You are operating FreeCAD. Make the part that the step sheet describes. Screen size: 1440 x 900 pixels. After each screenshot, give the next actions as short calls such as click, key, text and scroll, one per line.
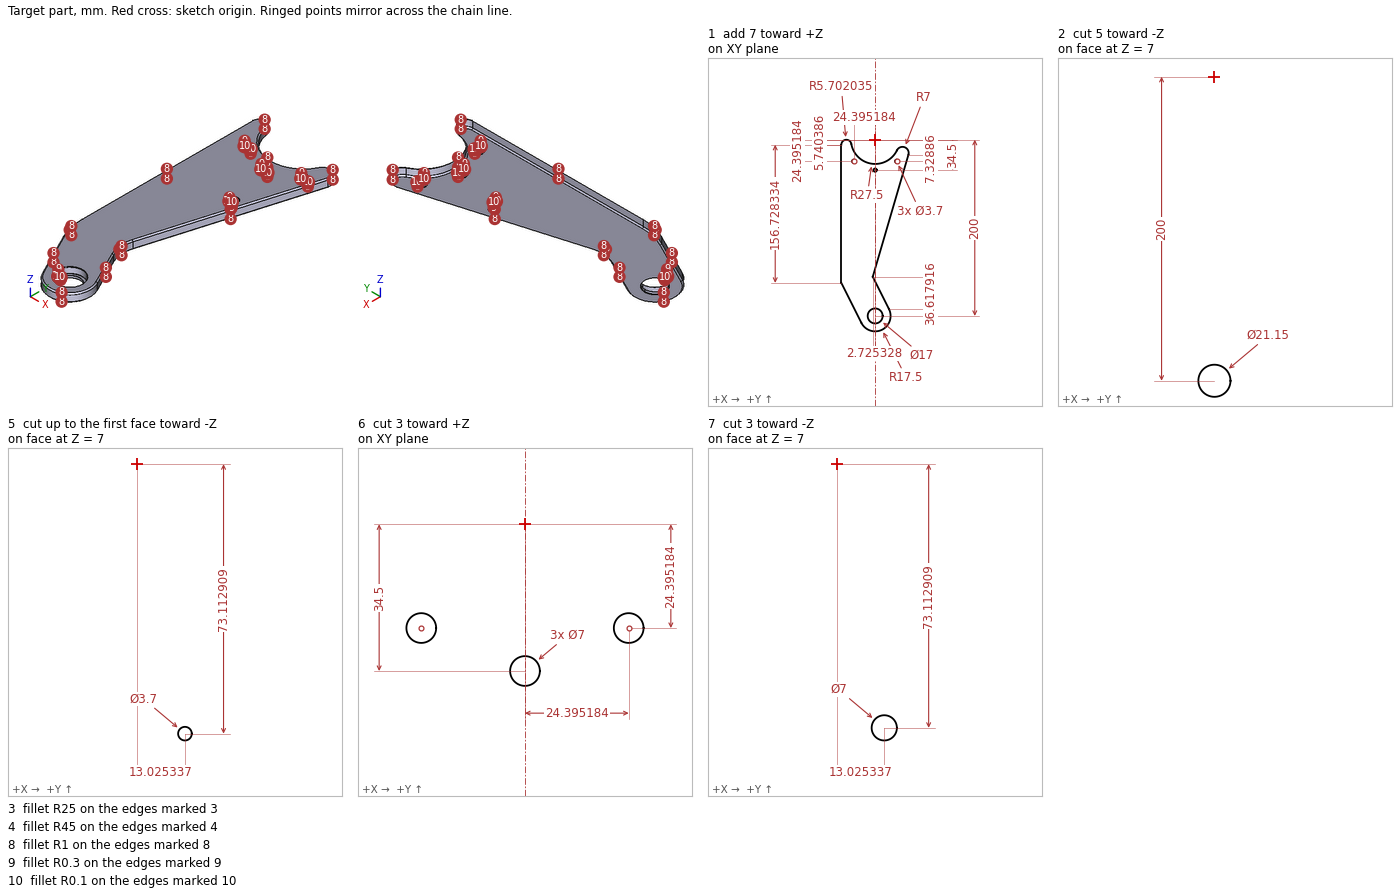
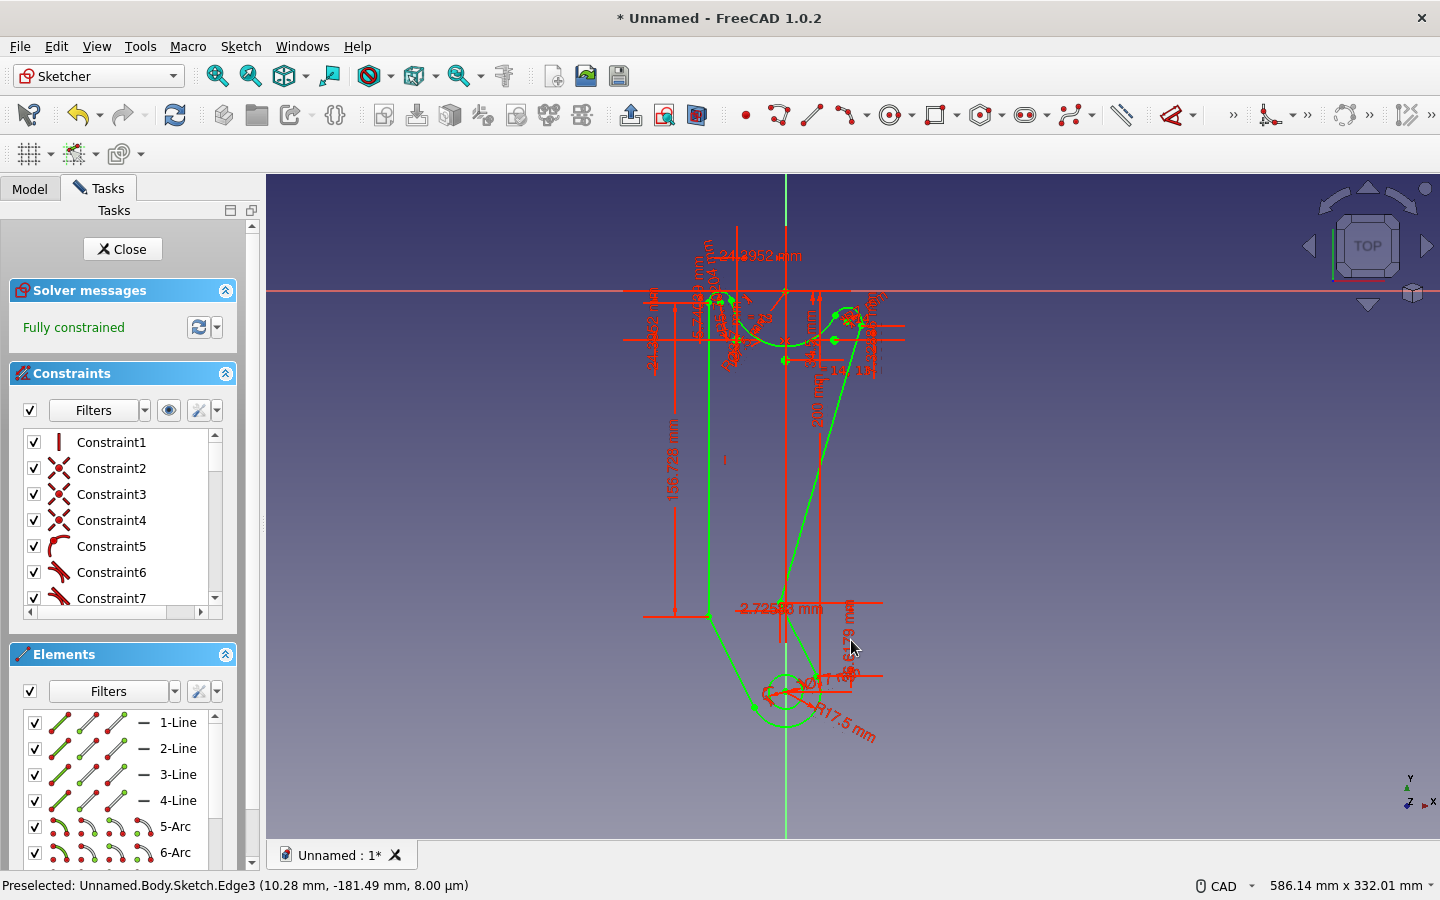
click(123, 249)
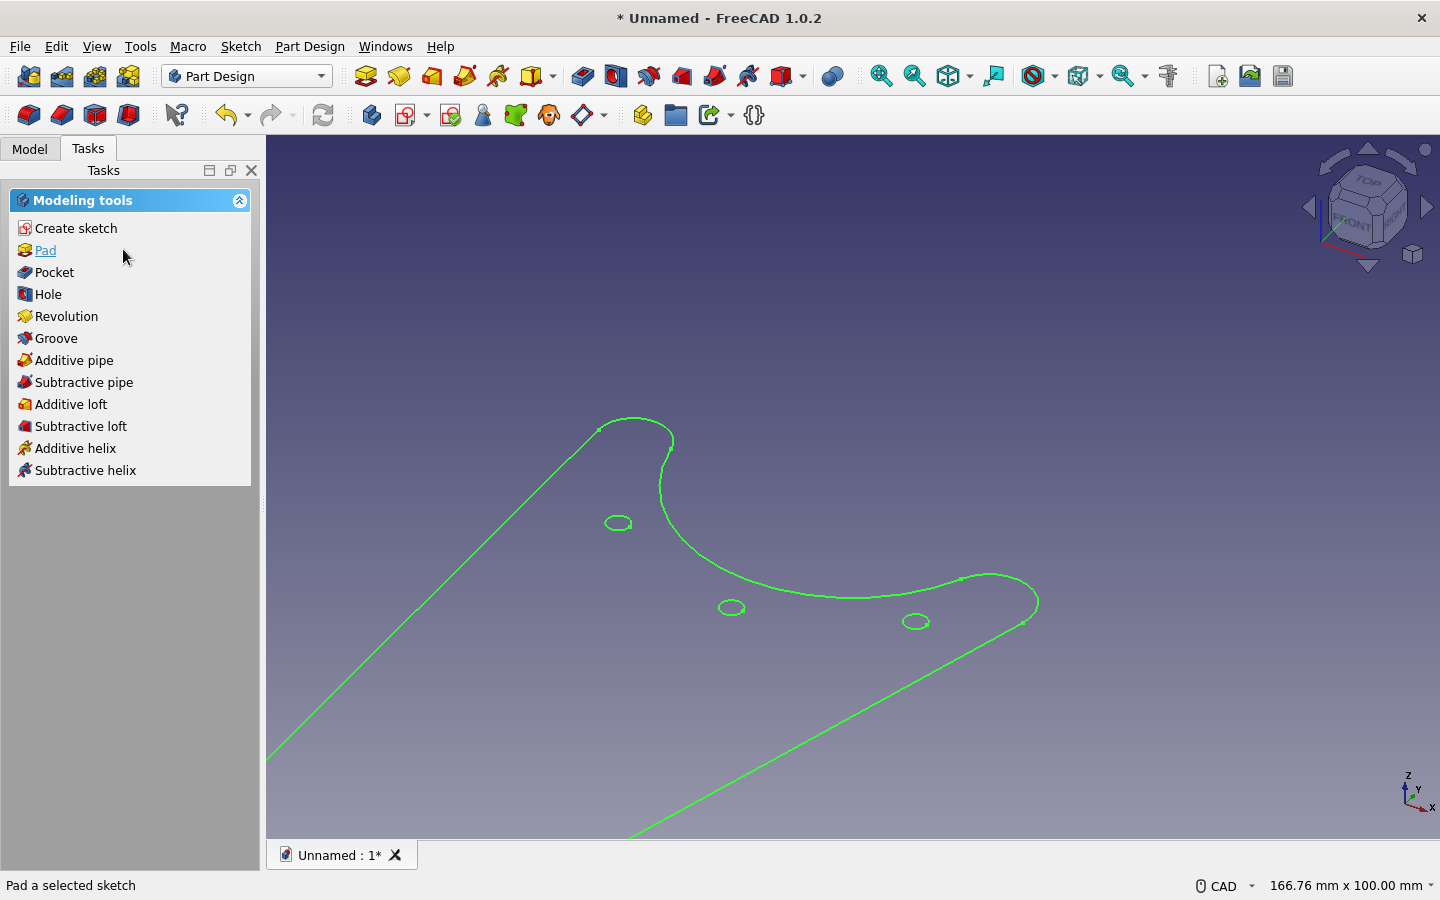
click(366, 76)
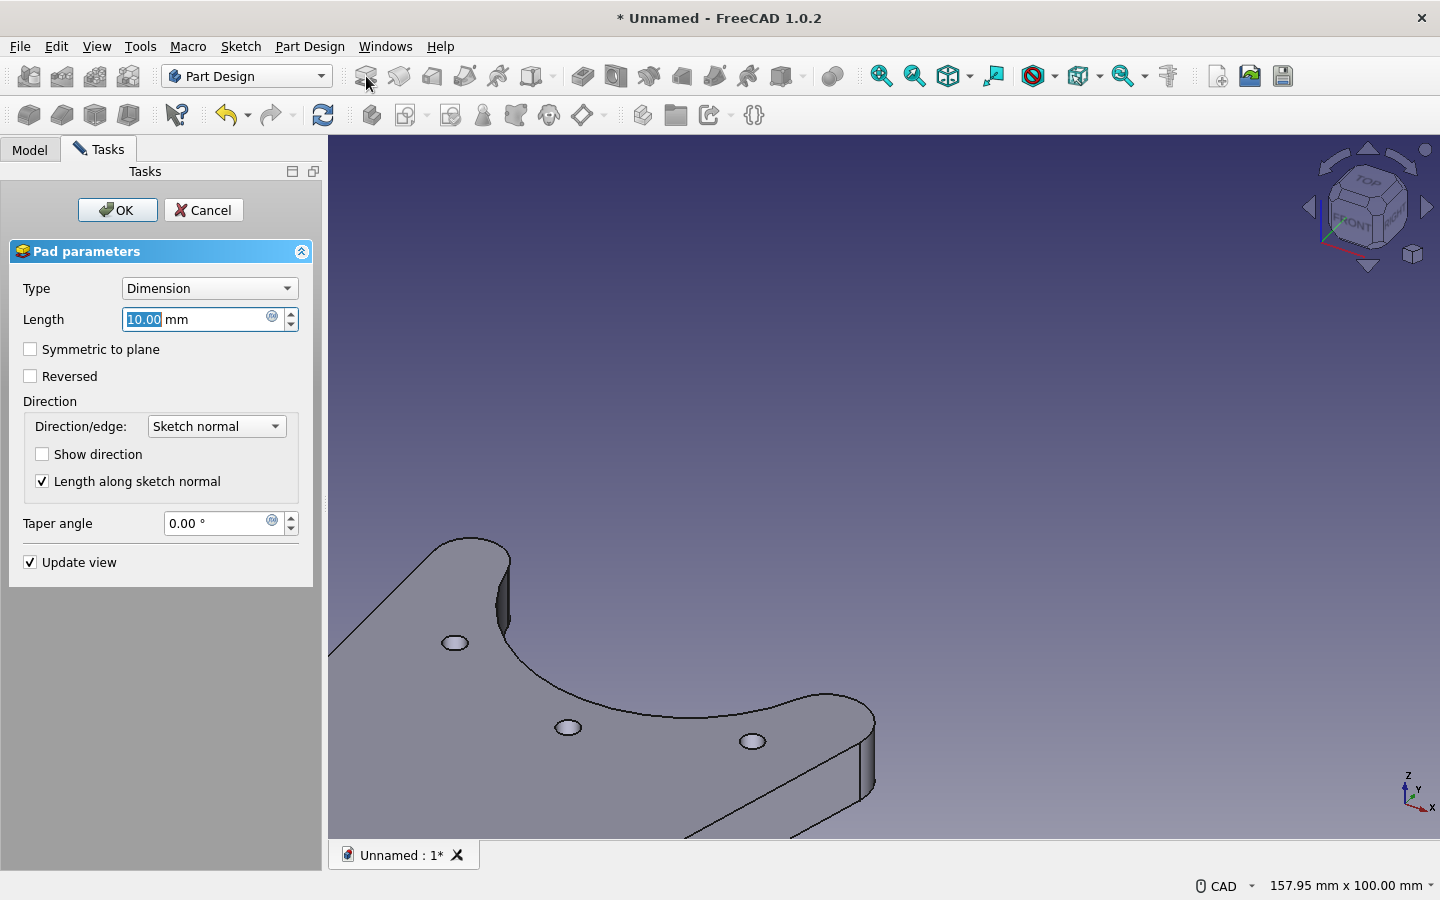
text(7)
key(Tab)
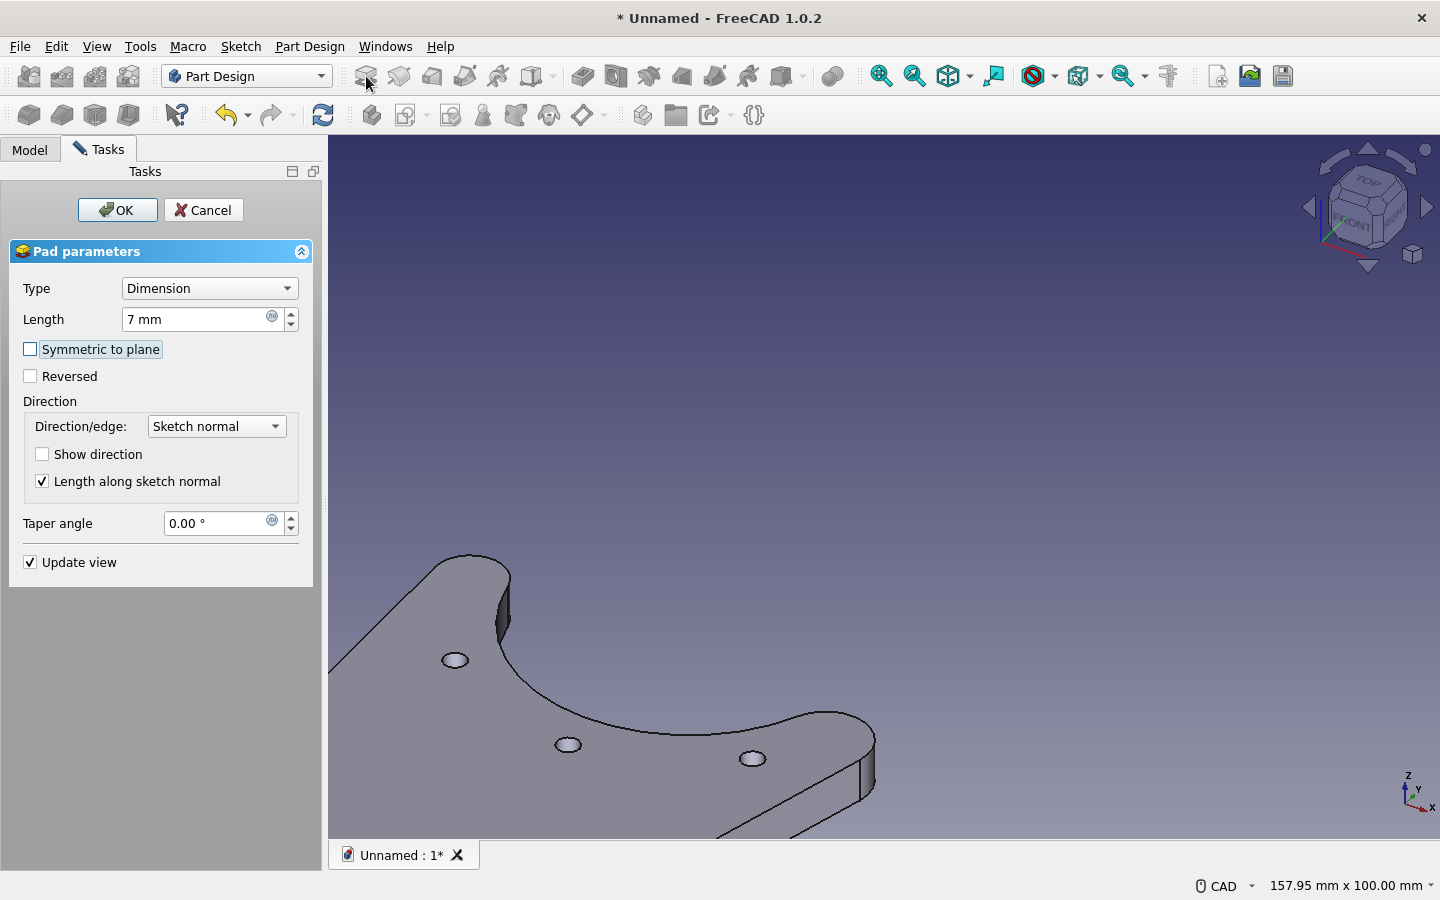
click(118, 210)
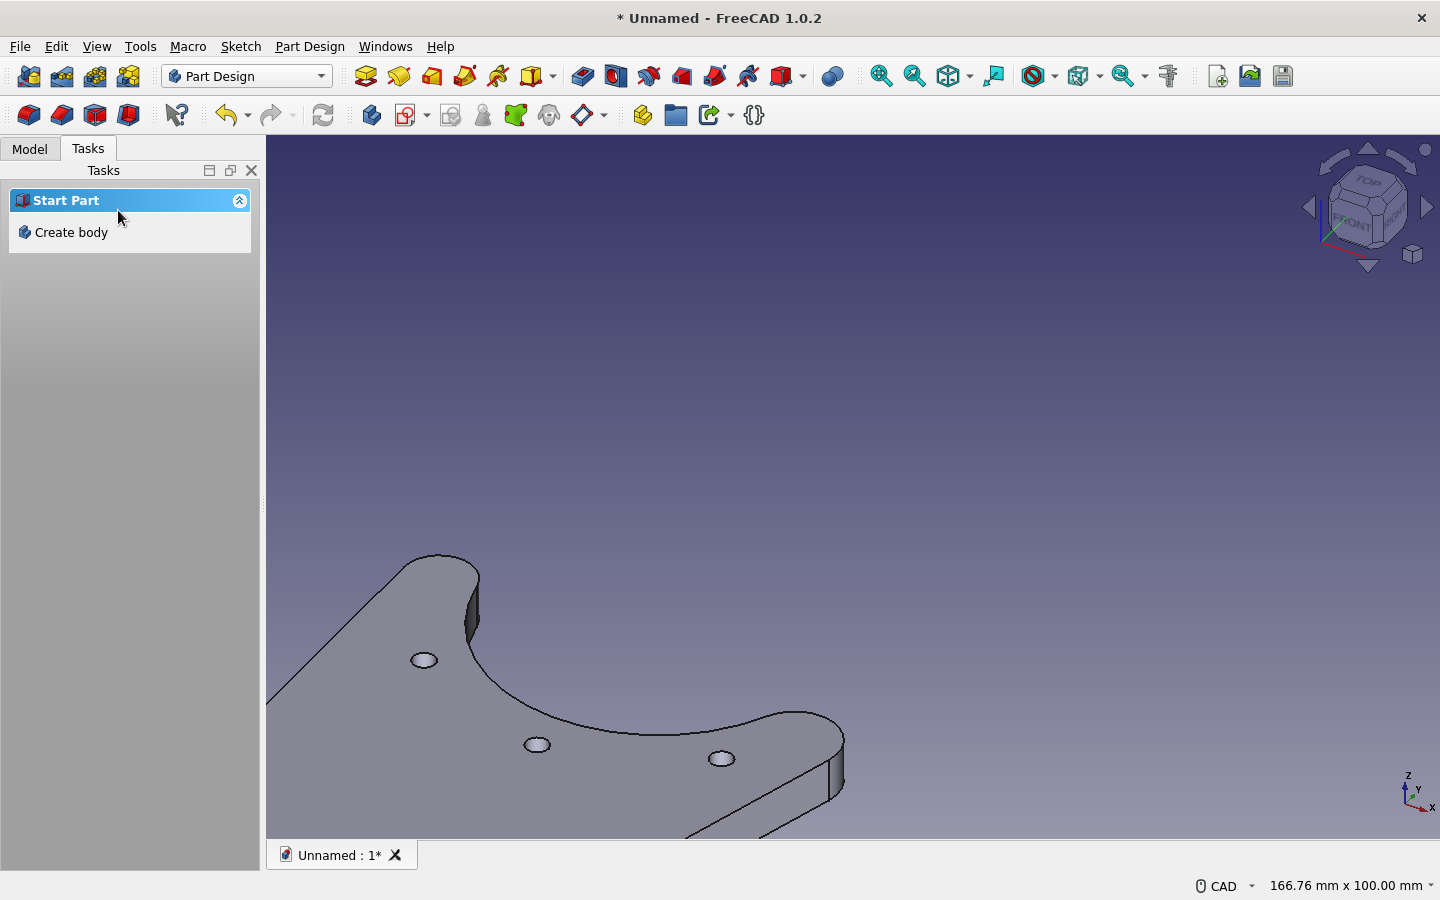
click(882, 76)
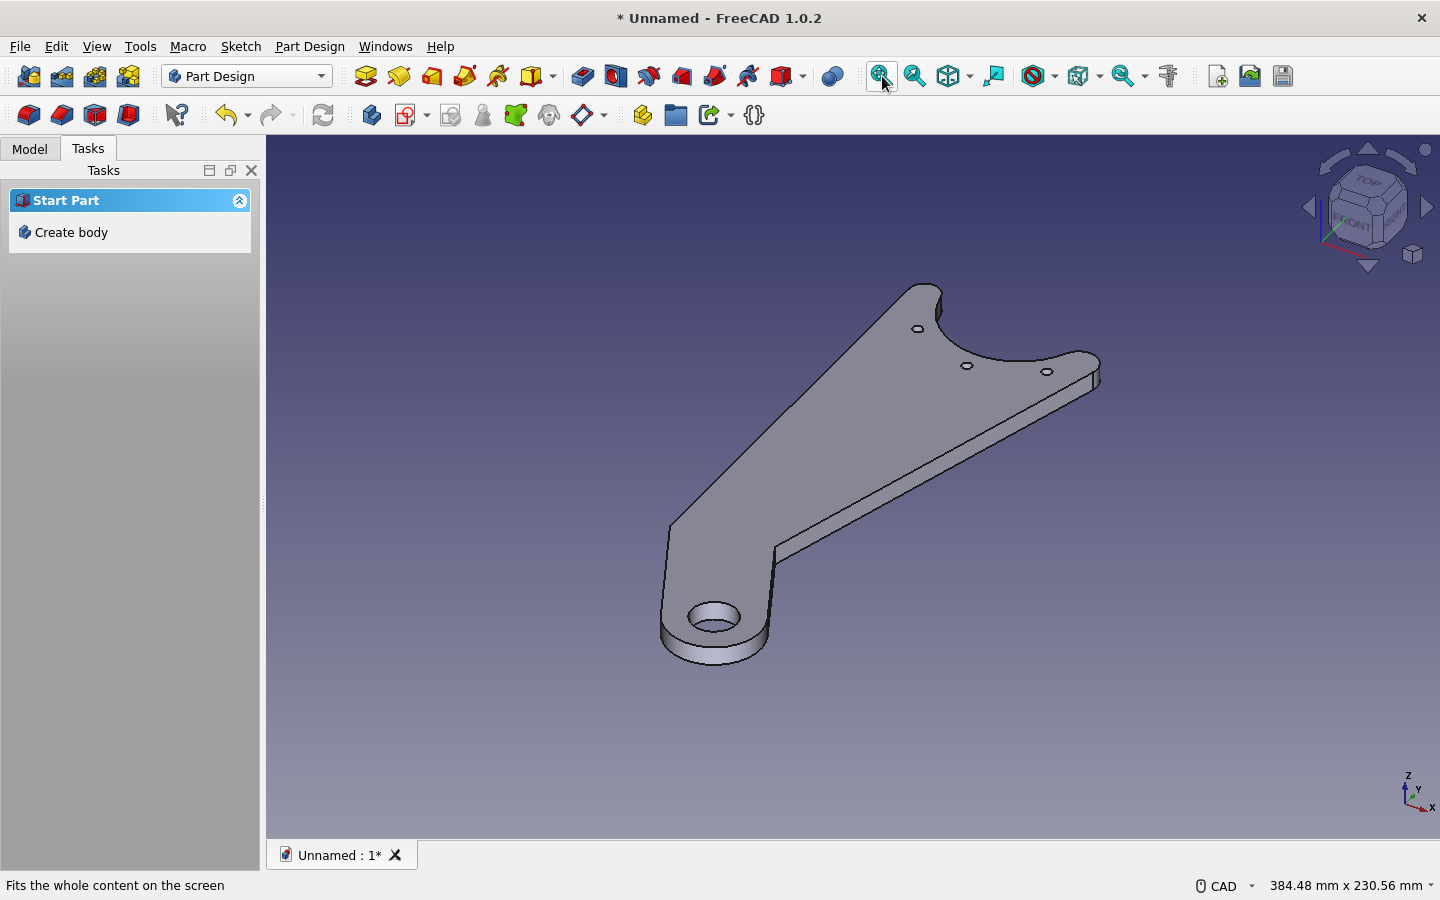
click(872, 421)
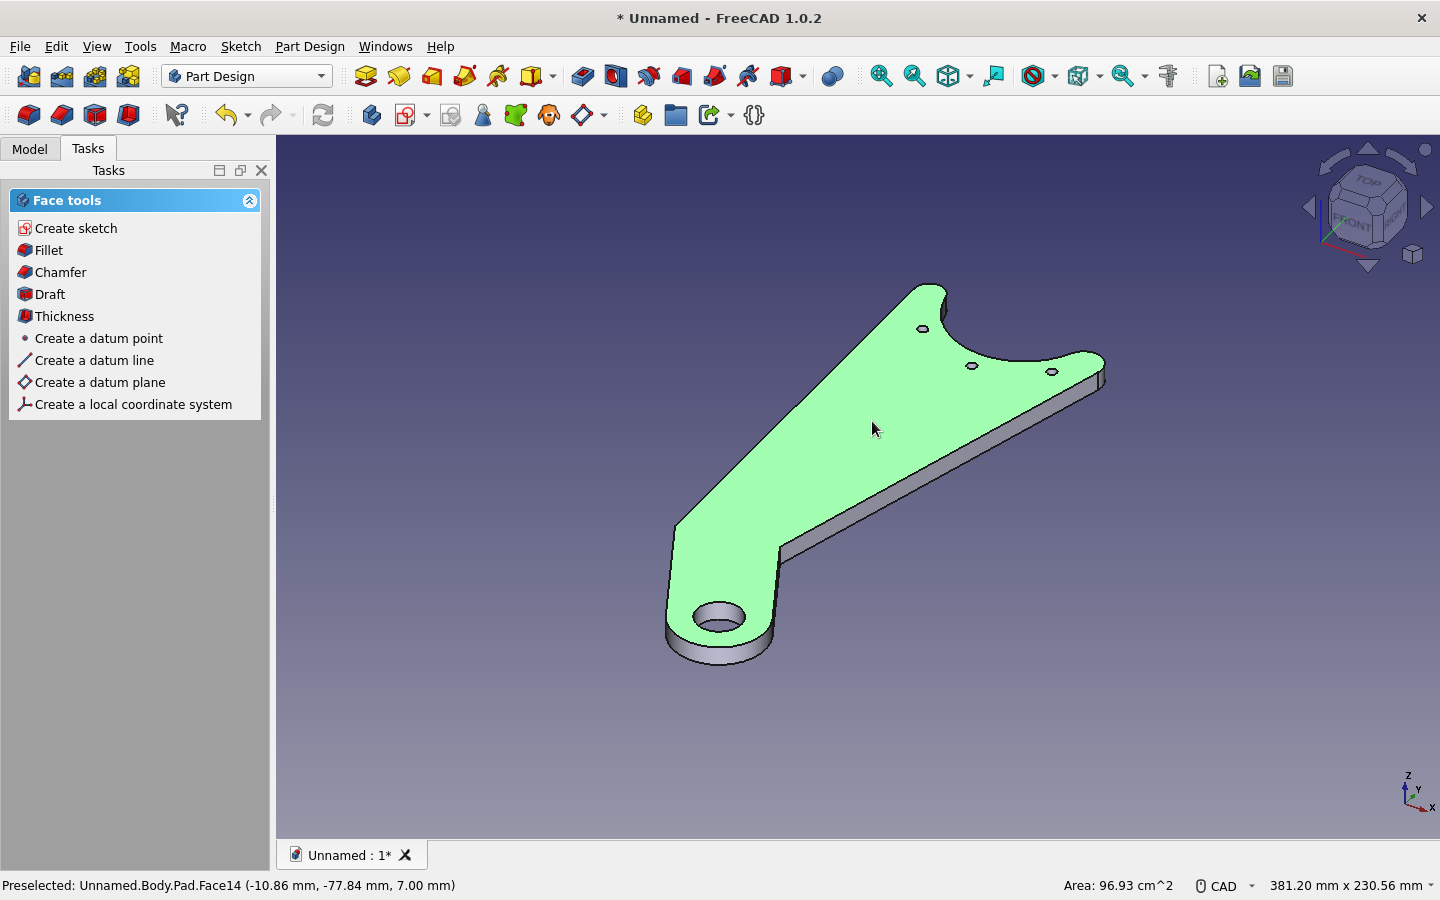
click(404, 116)